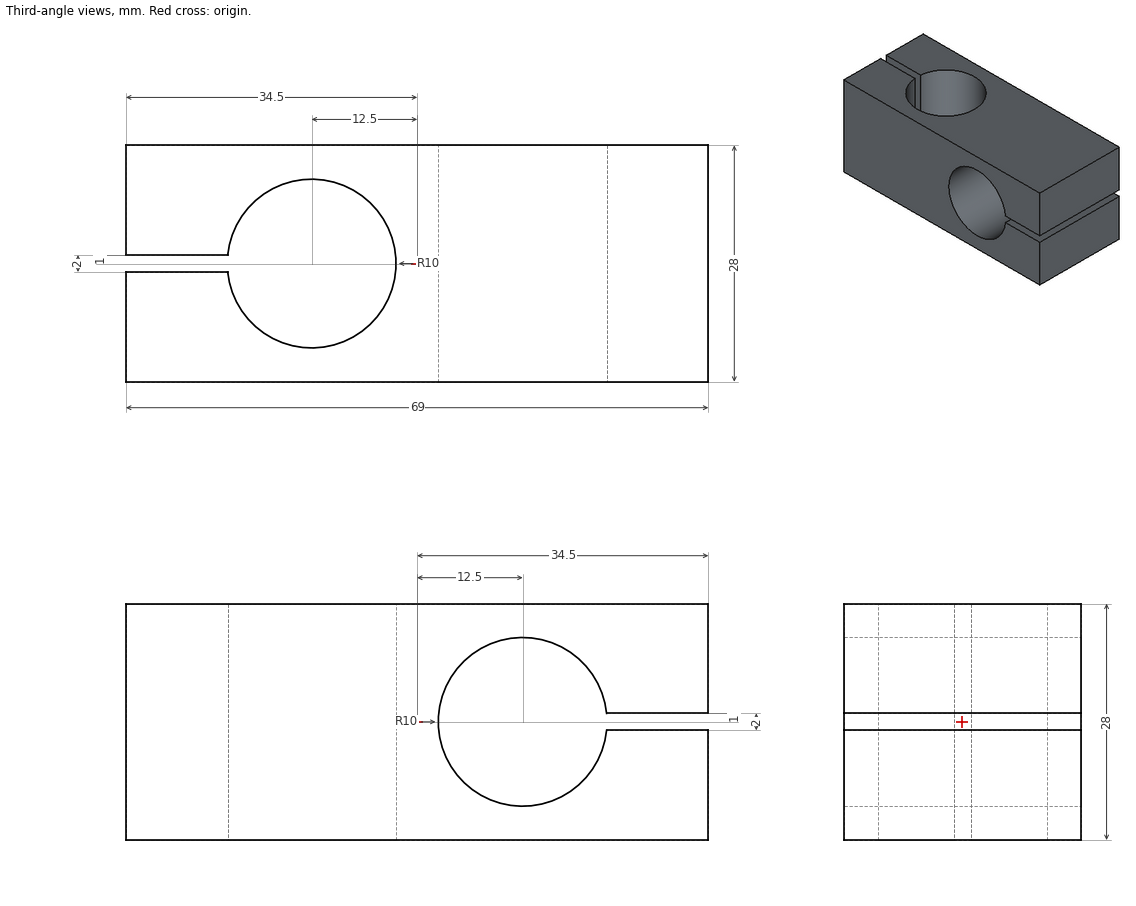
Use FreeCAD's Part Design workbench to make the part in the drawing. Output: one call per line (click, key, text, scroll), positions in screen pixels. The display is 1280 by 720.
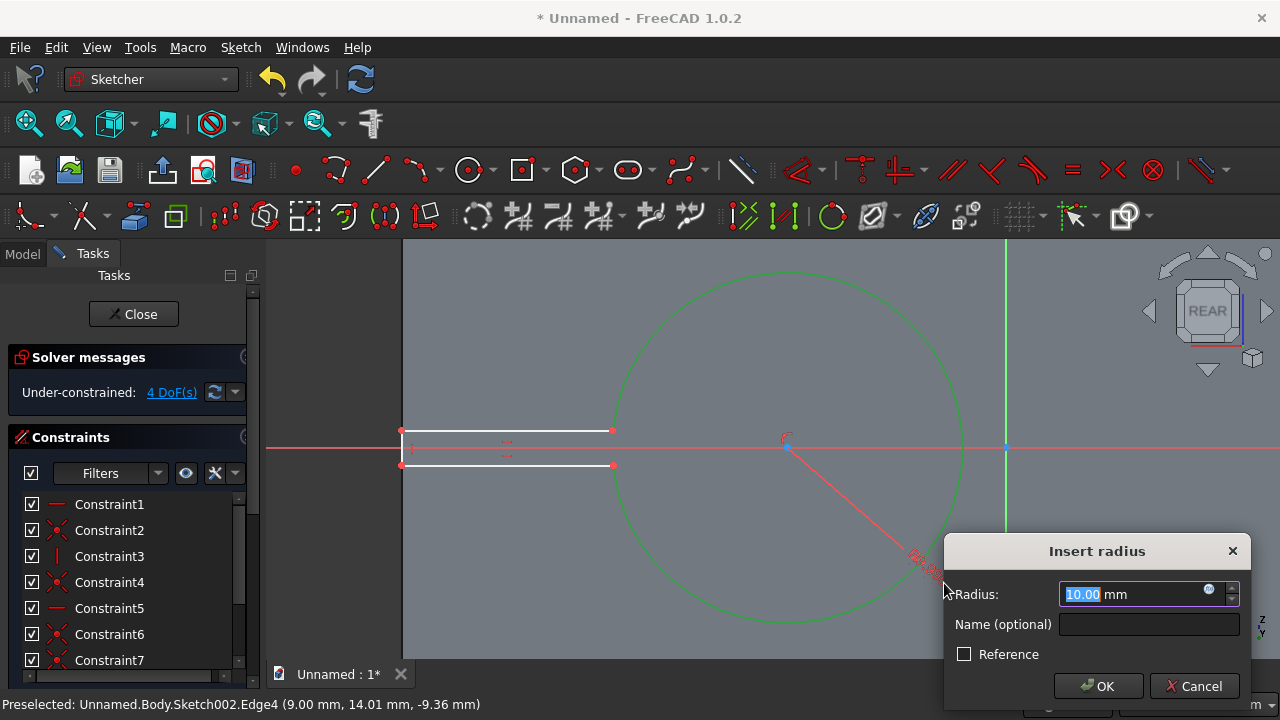
text(10)
key(Return)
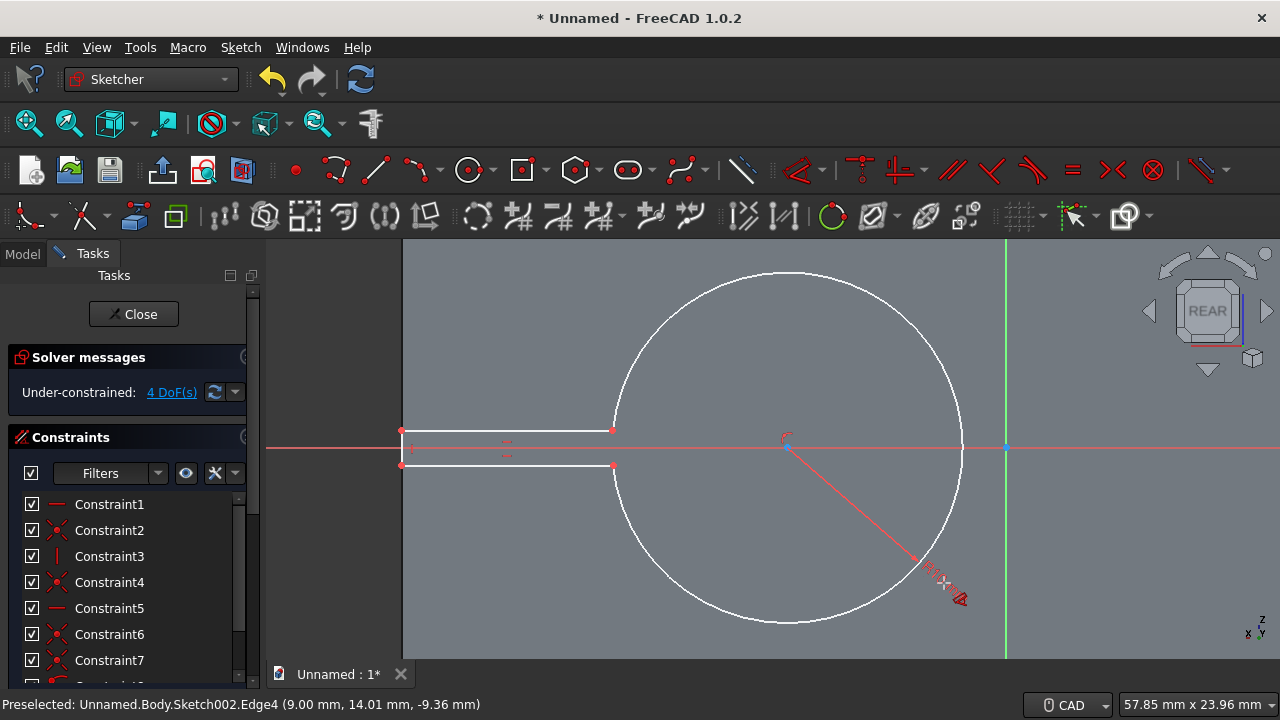
click(402, 445)
click(368, 440)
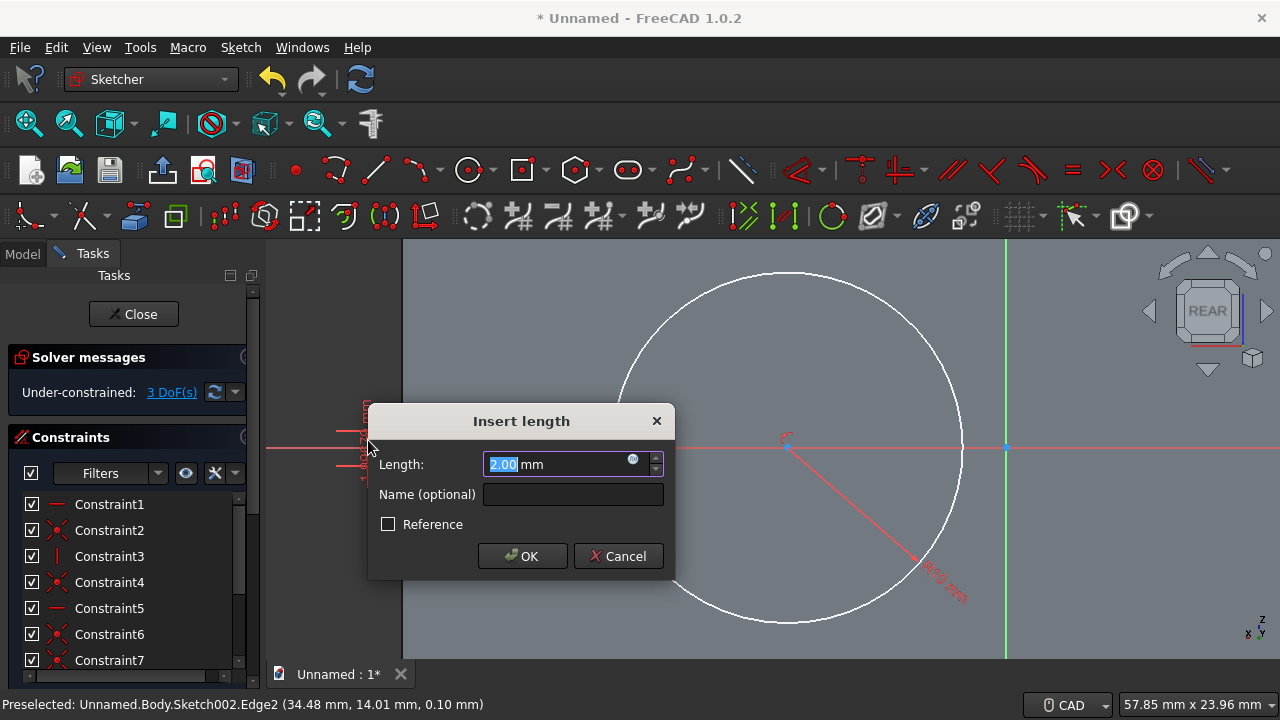
text(2)
key(Return)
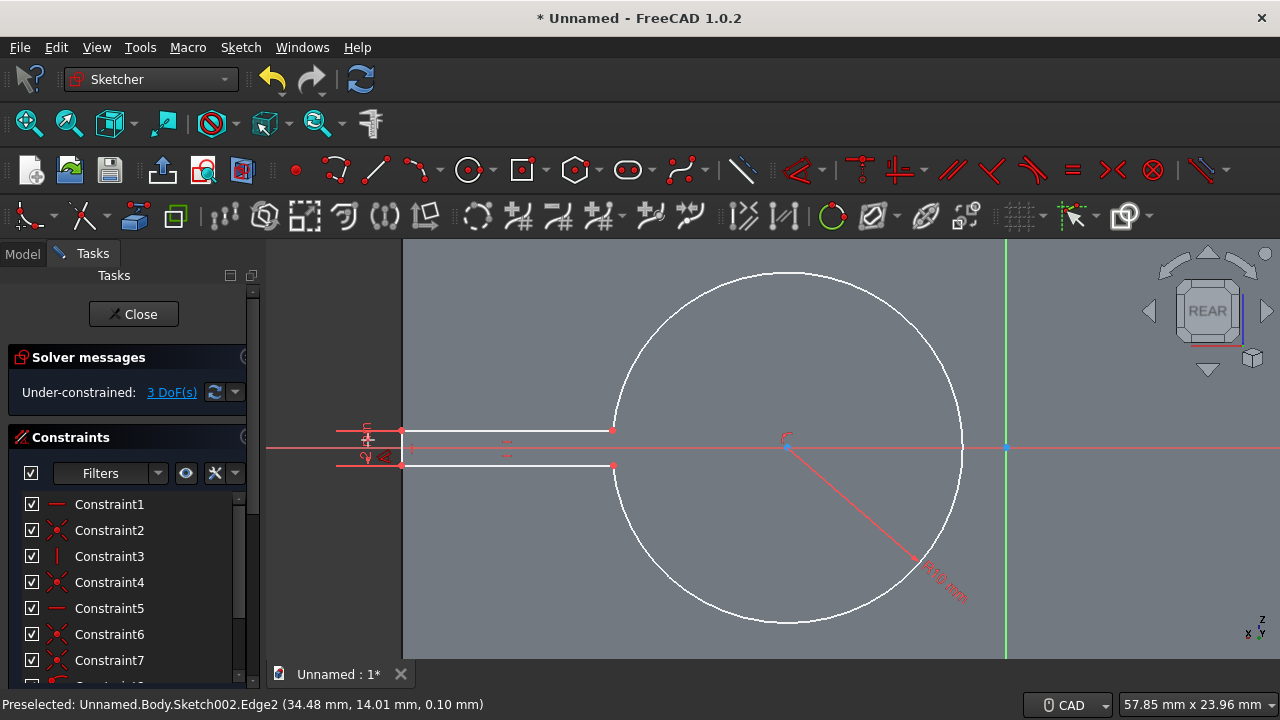
scroll(613, 431, up, 5)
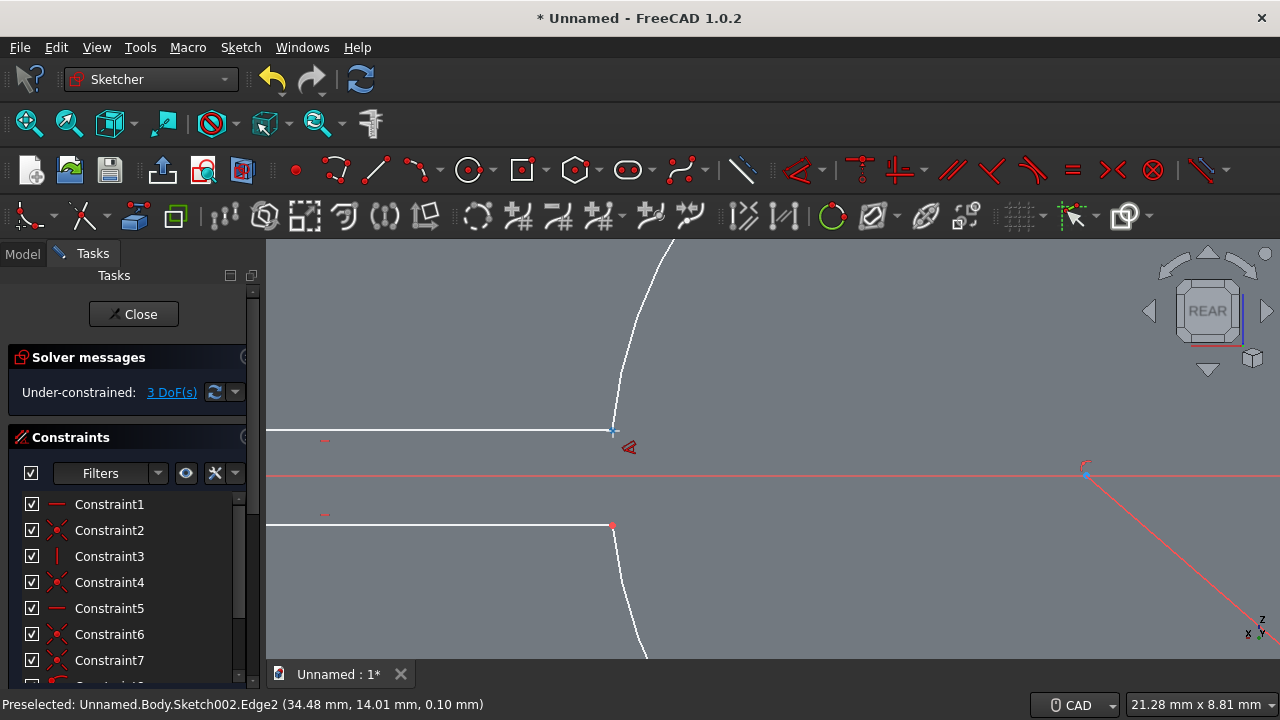
click(612, 430)
click(578, 453)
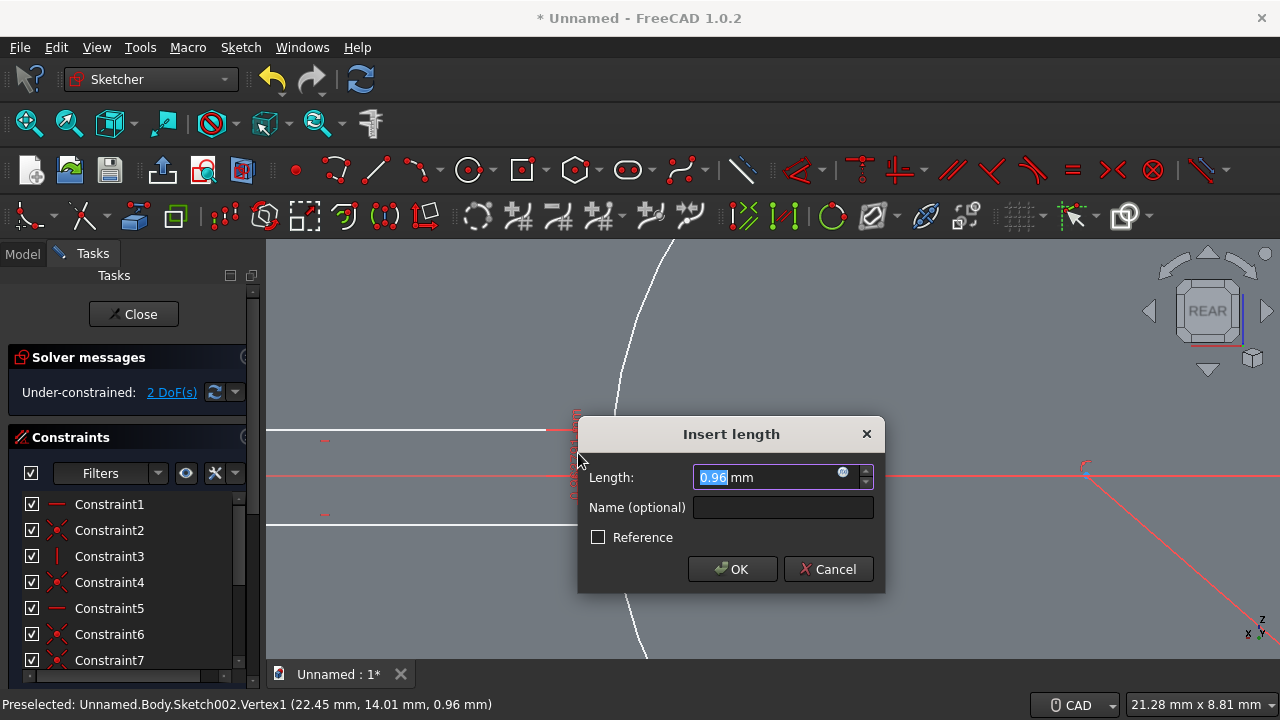
text(1)
key(Return)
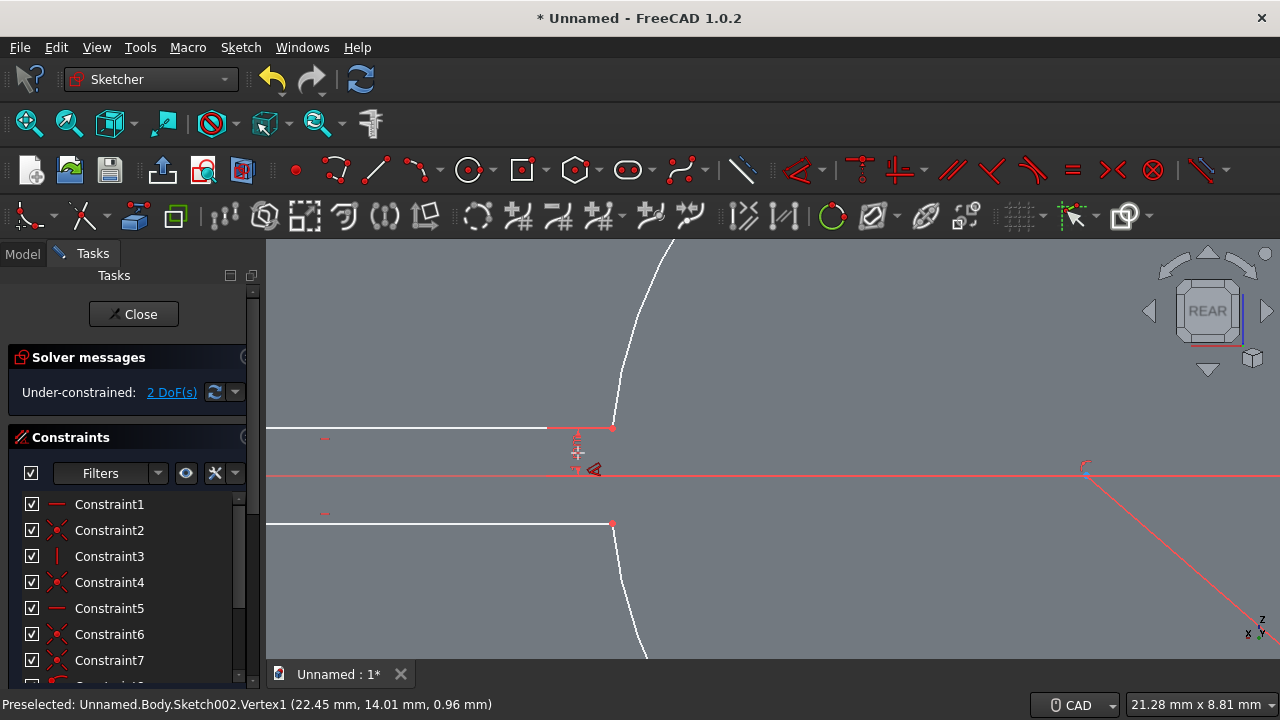
scroll(614, 433, down, 5)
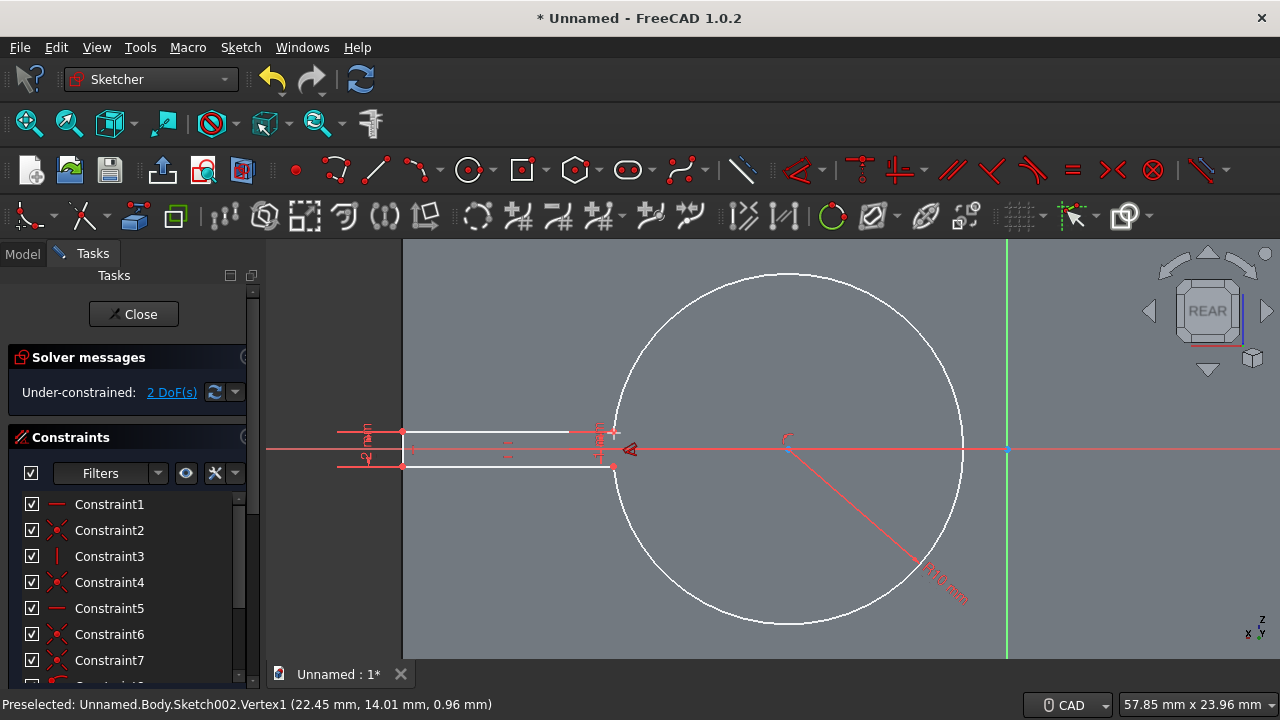
click(403, 432)
click(705, 398)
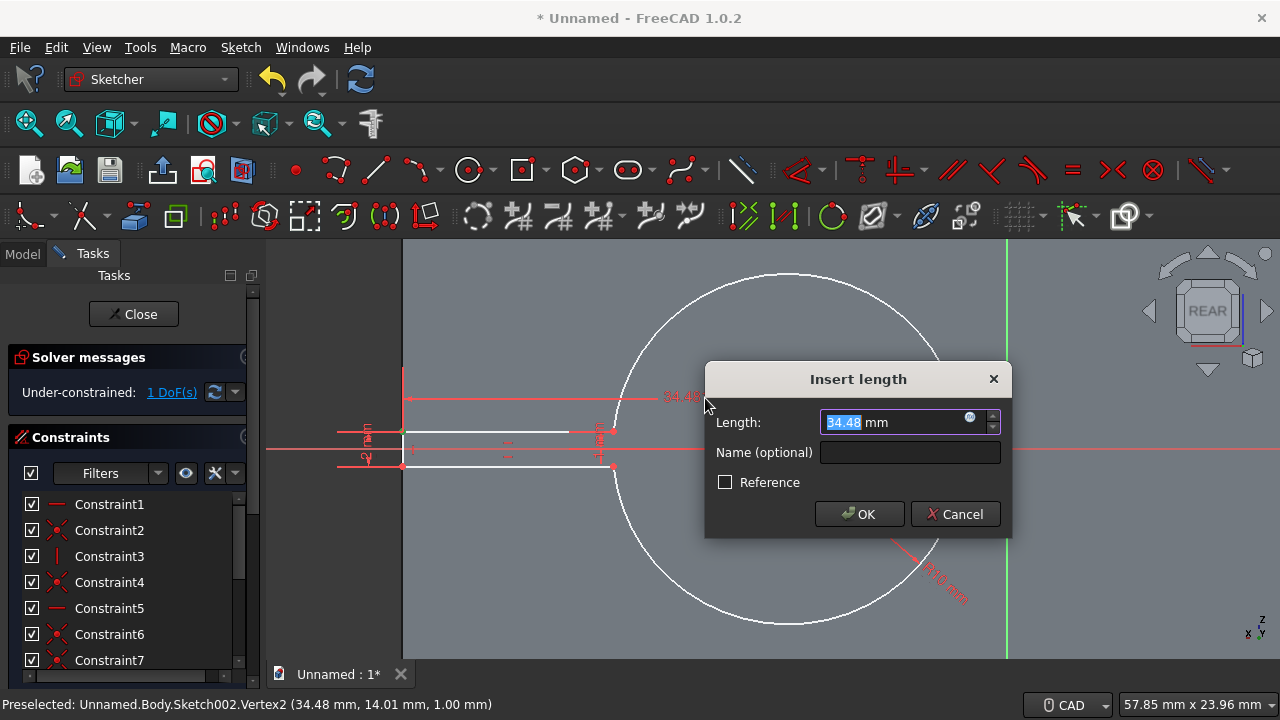
text(34.5)
key(Return)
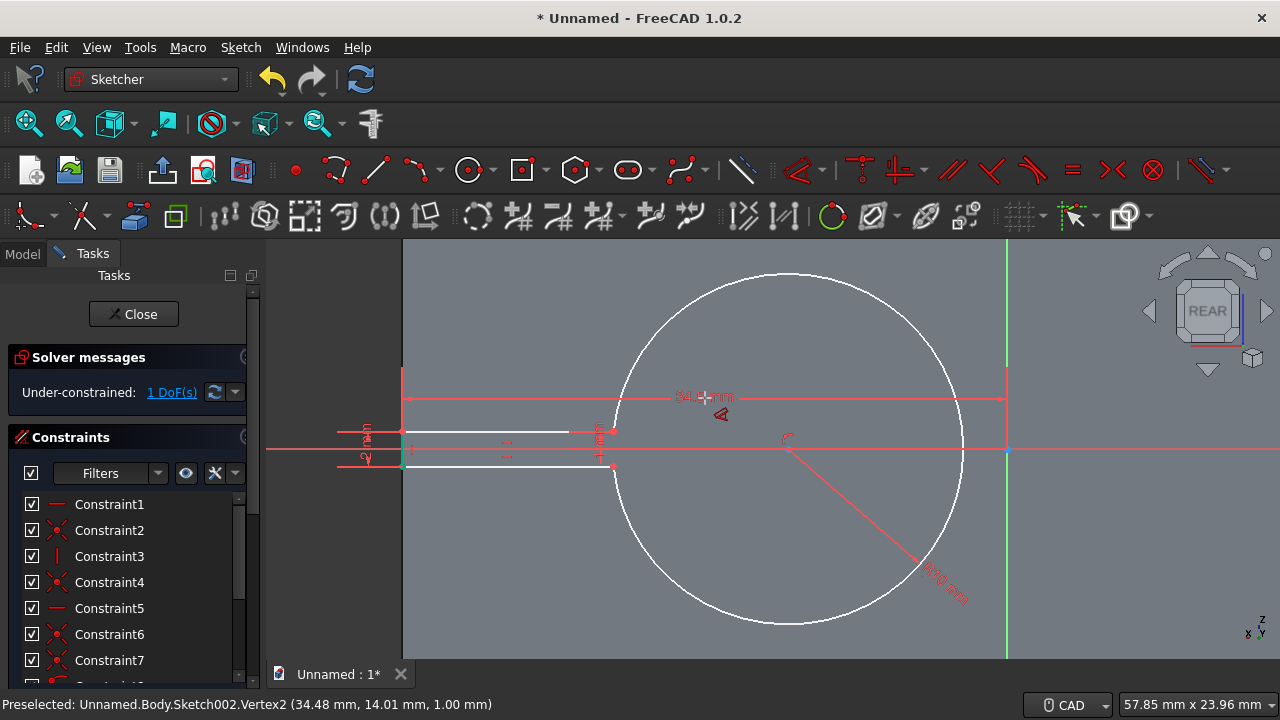
click(788, 449)
click(898, 483)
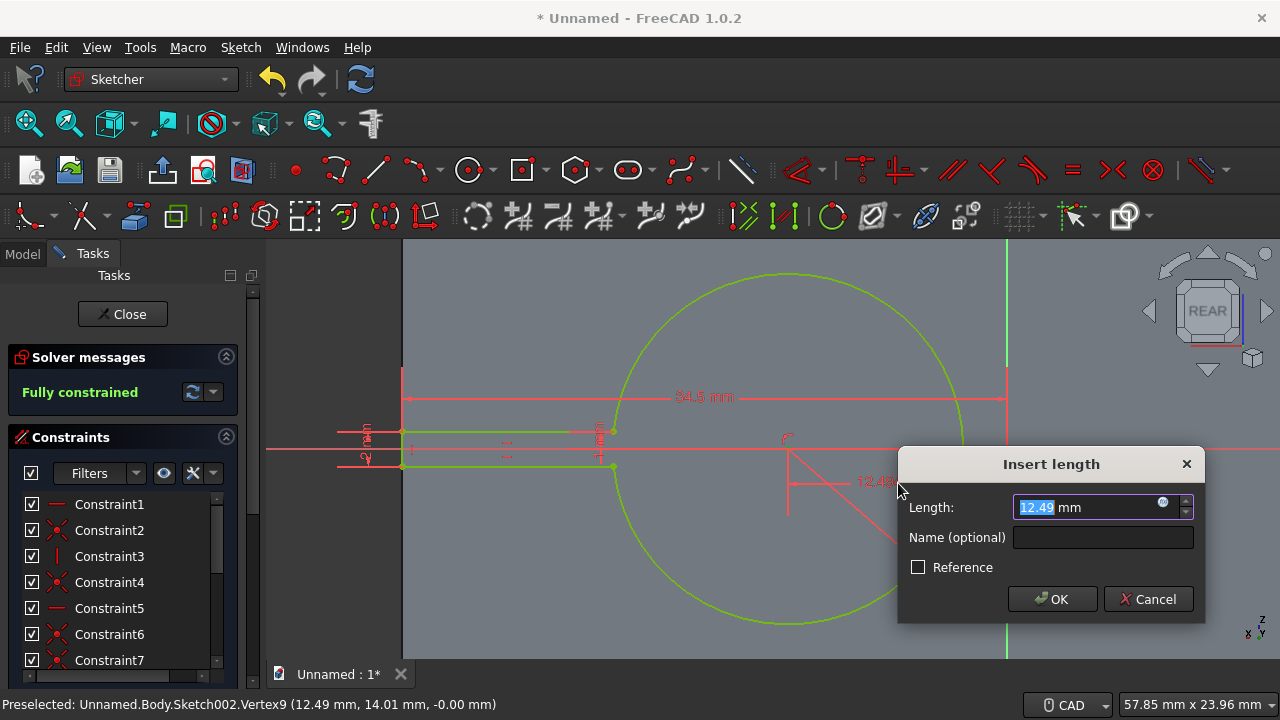
text(12.5)
key(Return)
key(Escape)